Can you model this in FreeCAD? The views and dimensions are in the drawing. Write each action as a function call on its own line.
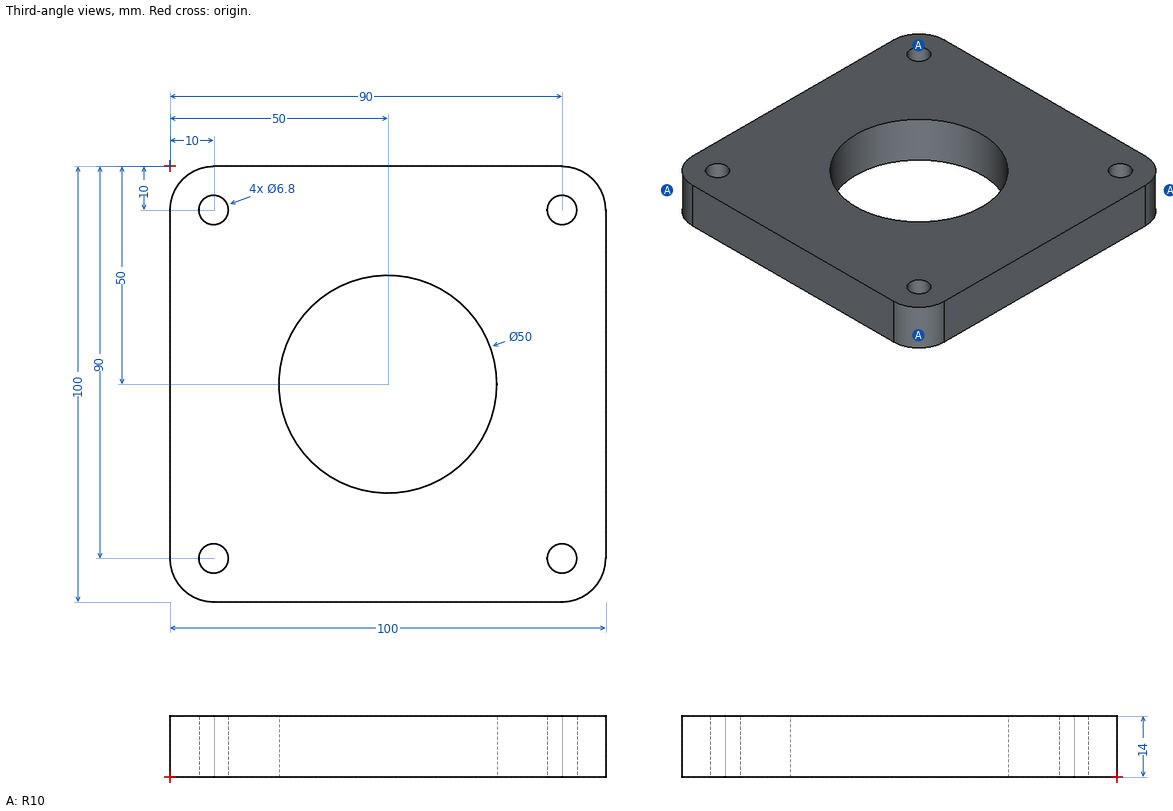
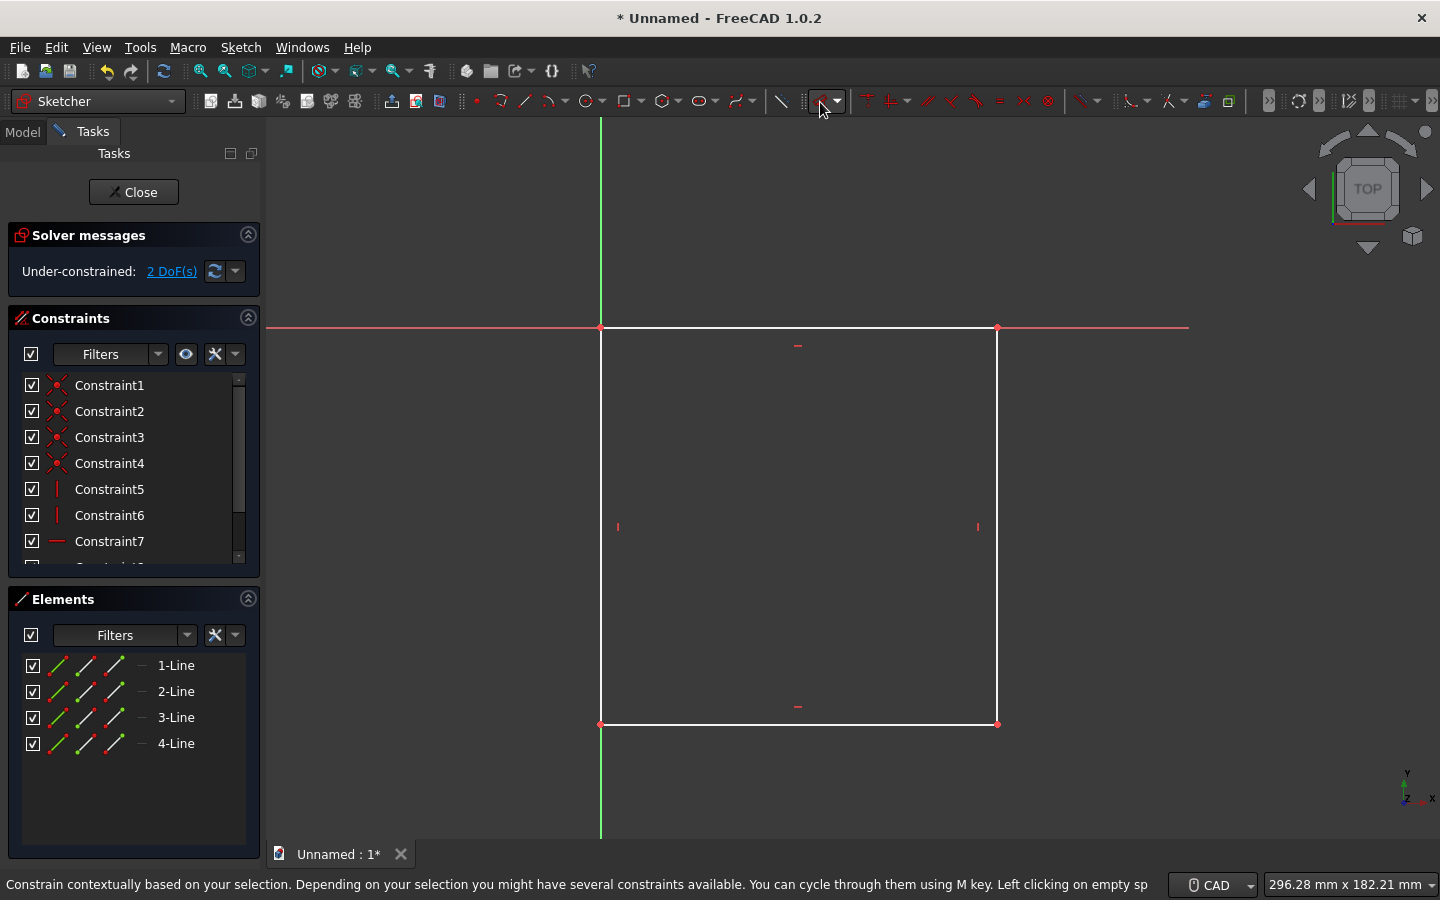
click(601, 447)
click(567, 526)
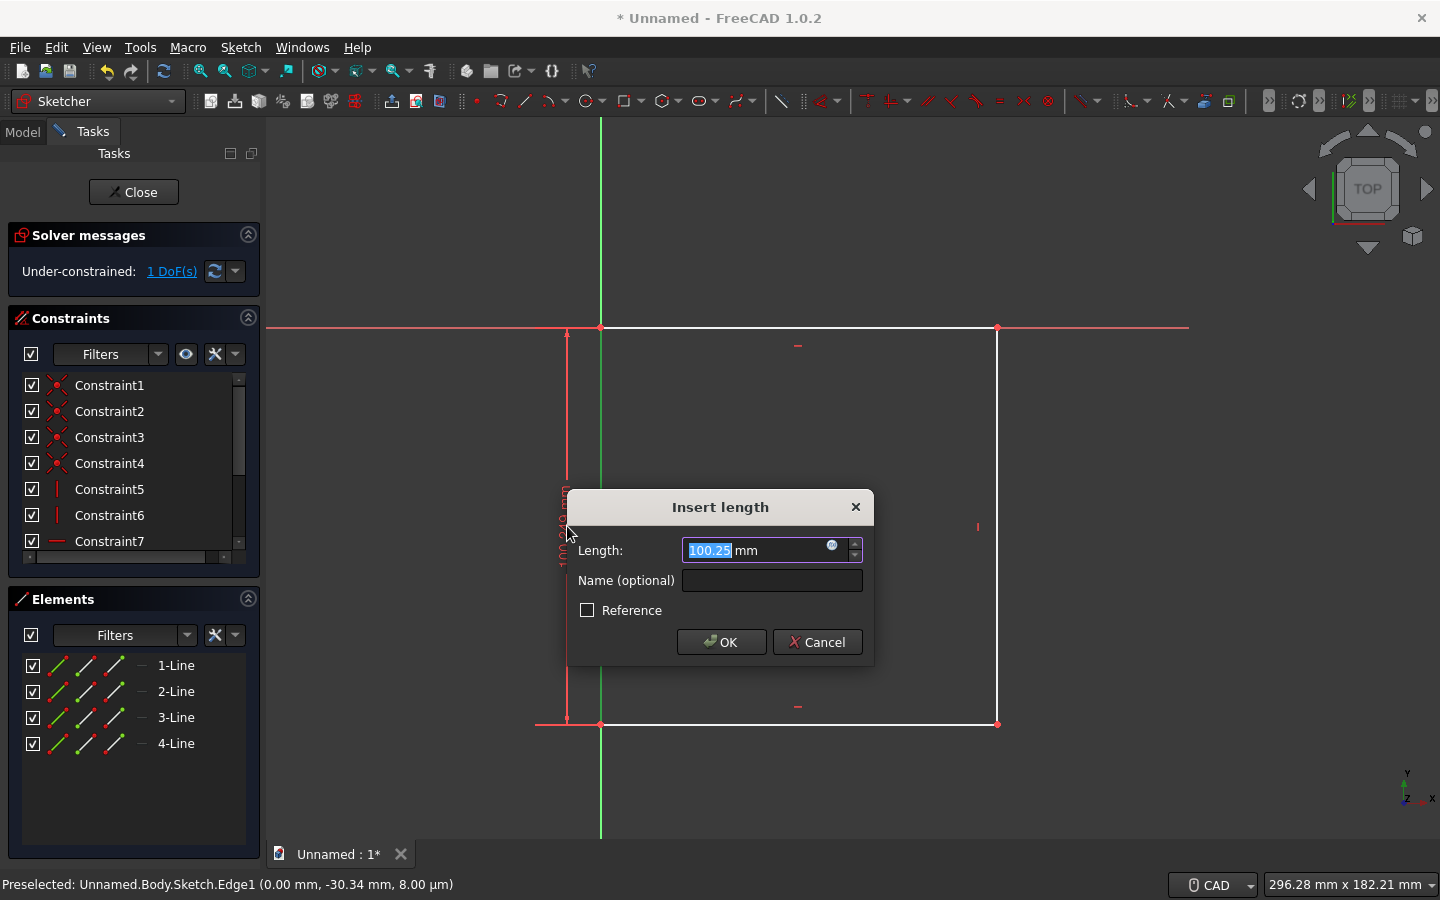
text(100)
key(Return)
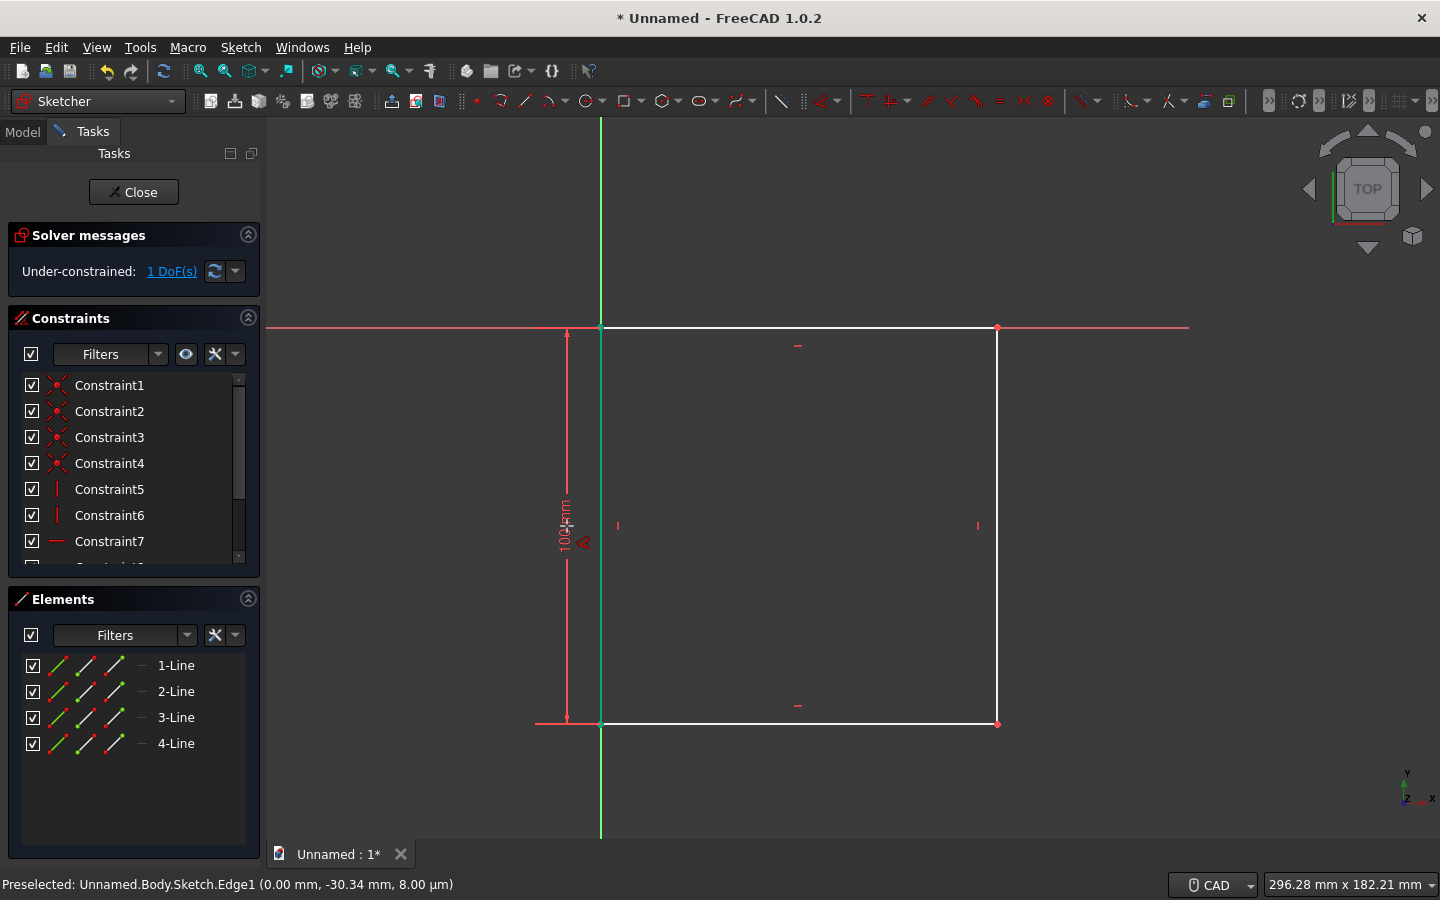
click(720, 724)
click(799, 758)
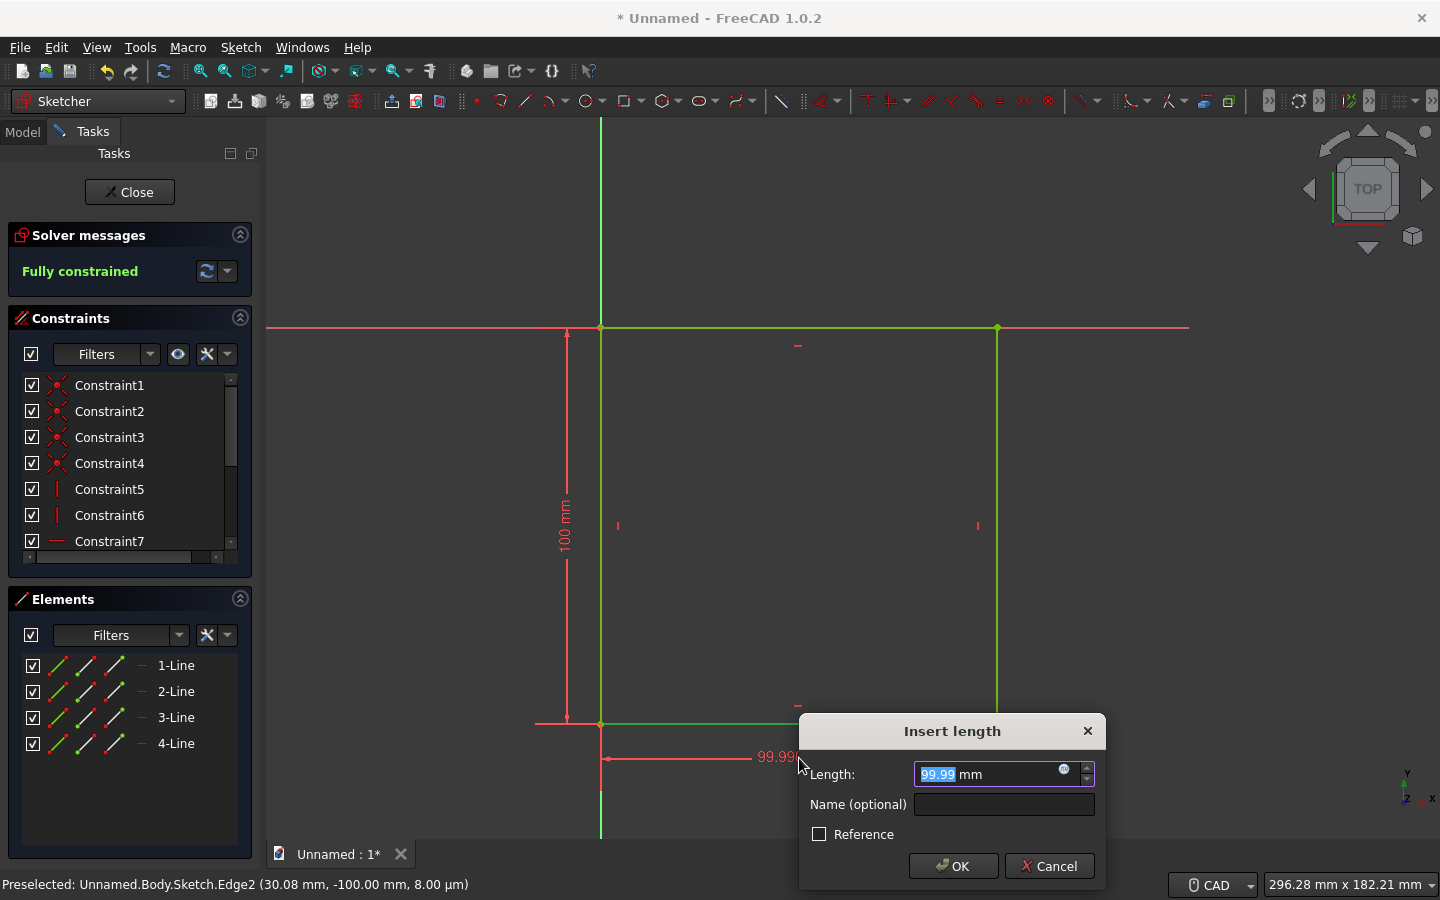
text(100)
key(Return)
key(Escape)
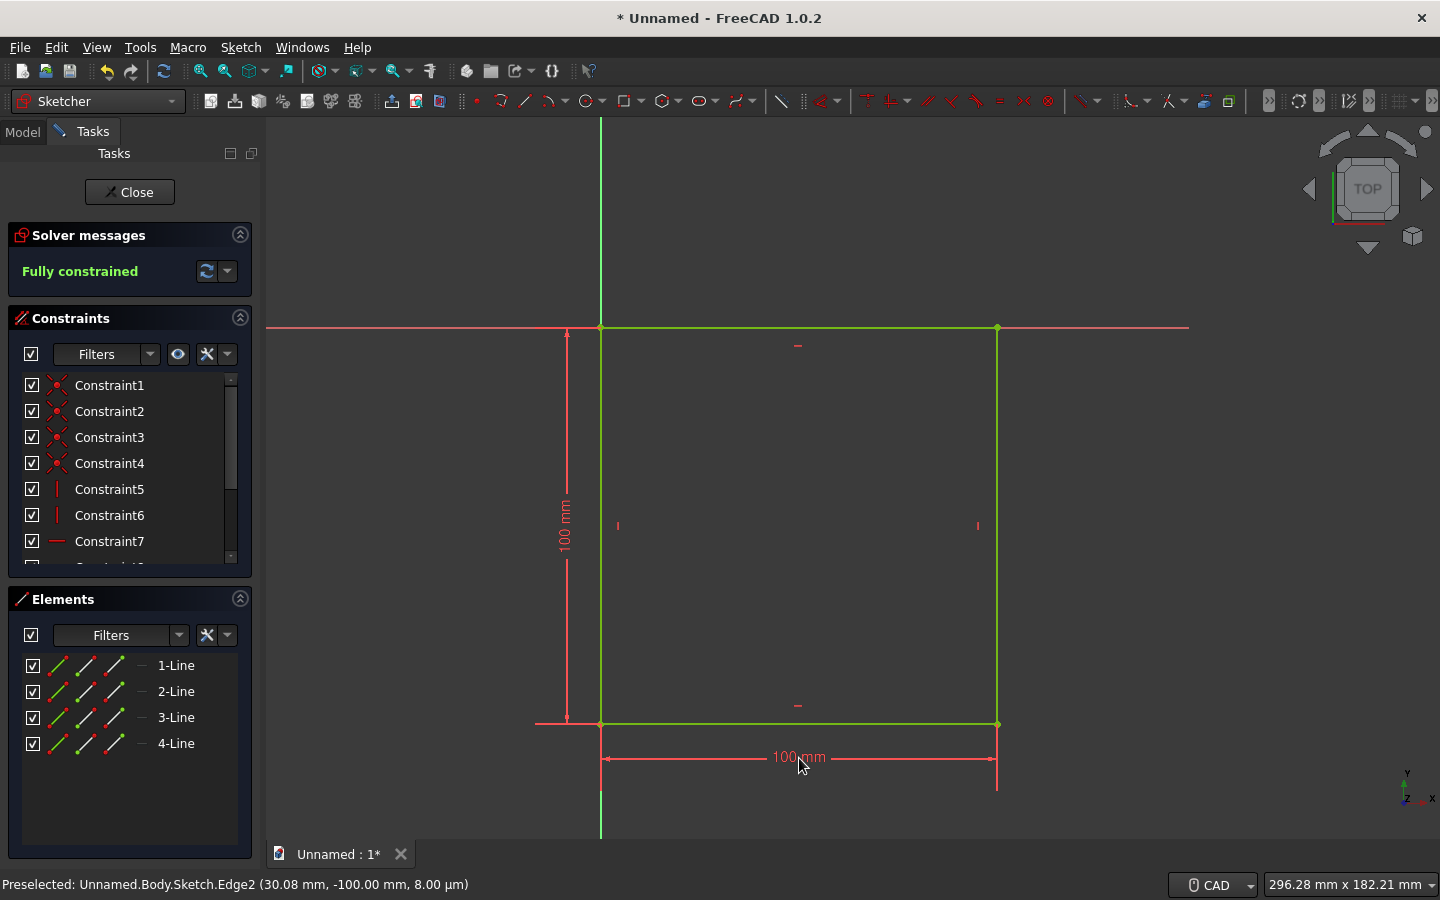
click(130, 192)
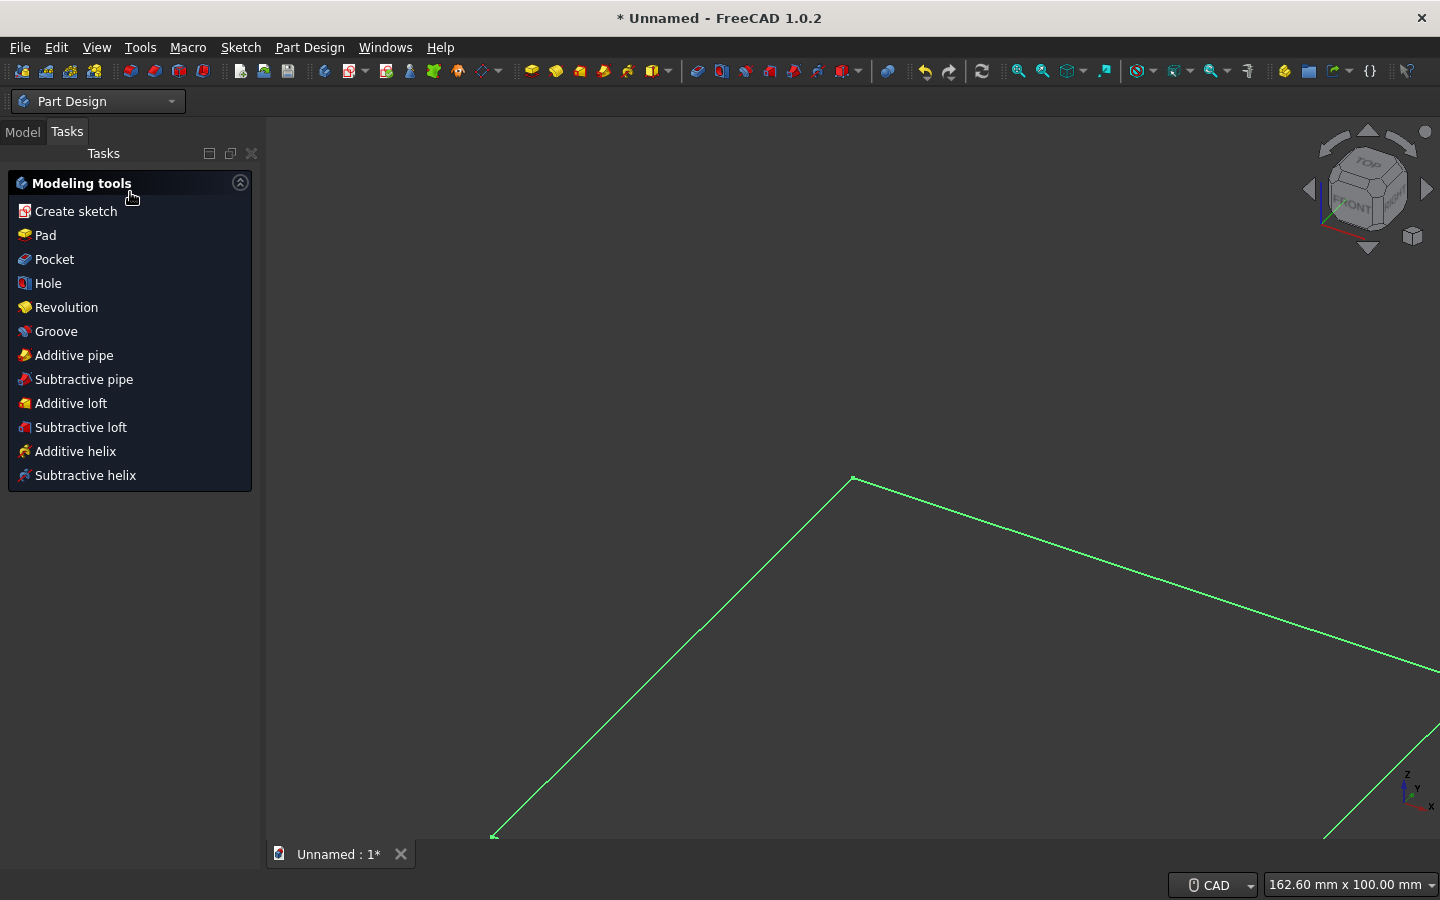
click(532, 72)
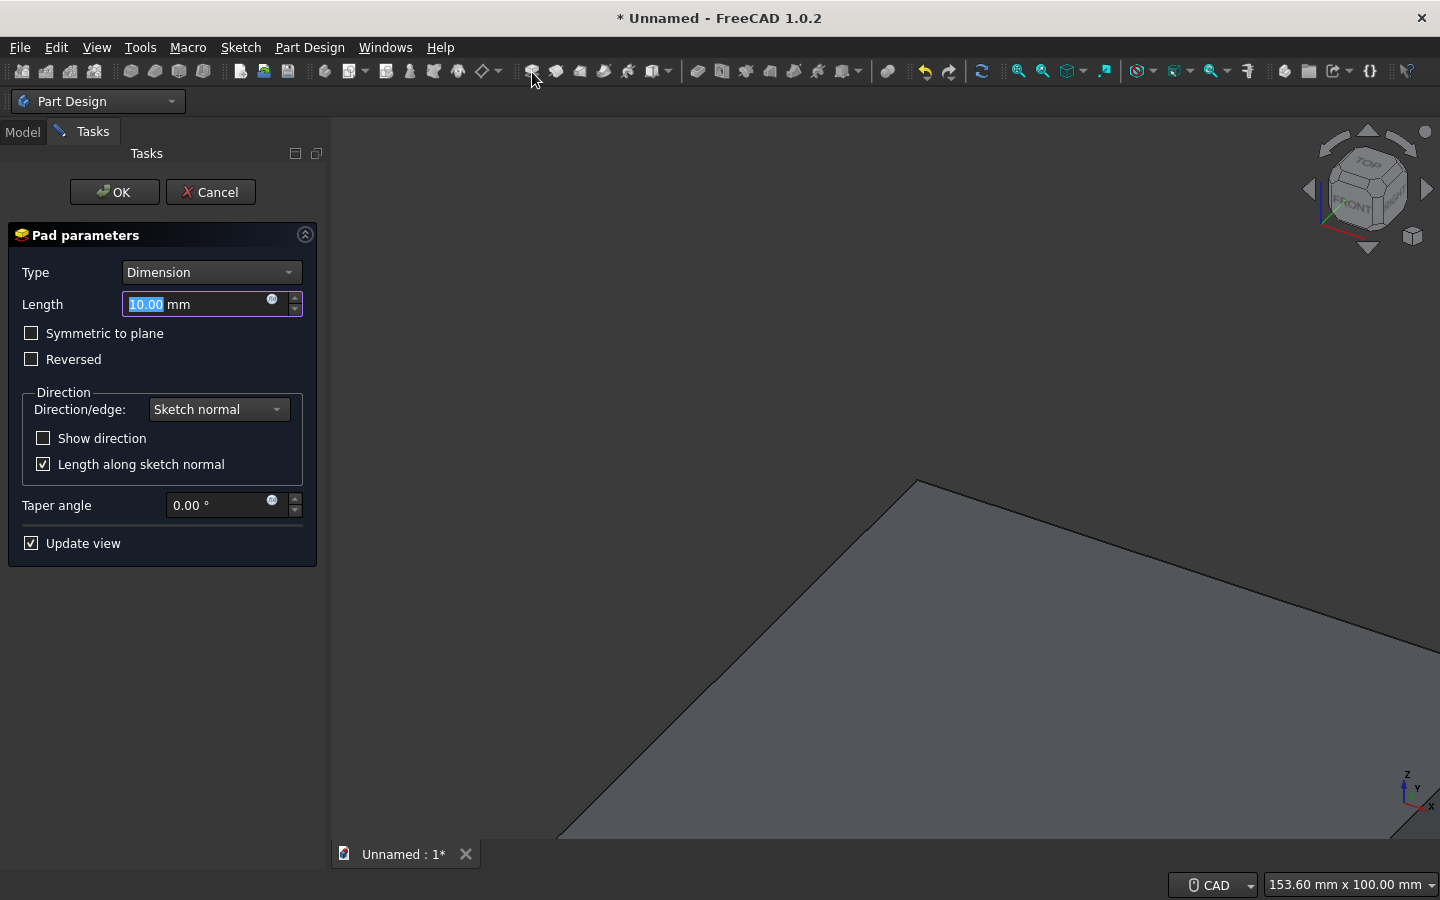
text(14)
key(Tab)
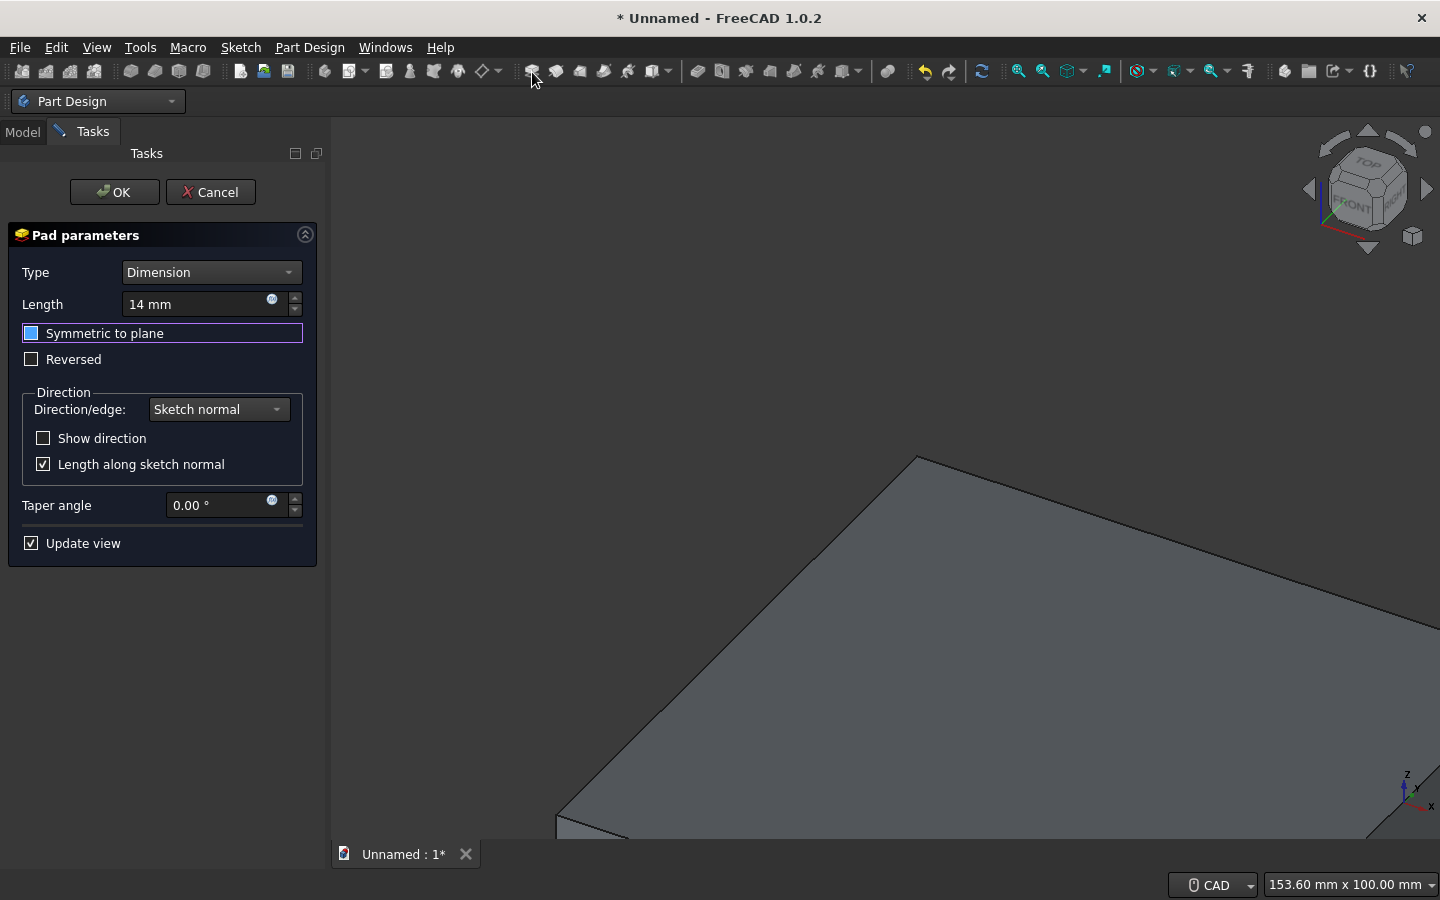
click(115, 192)